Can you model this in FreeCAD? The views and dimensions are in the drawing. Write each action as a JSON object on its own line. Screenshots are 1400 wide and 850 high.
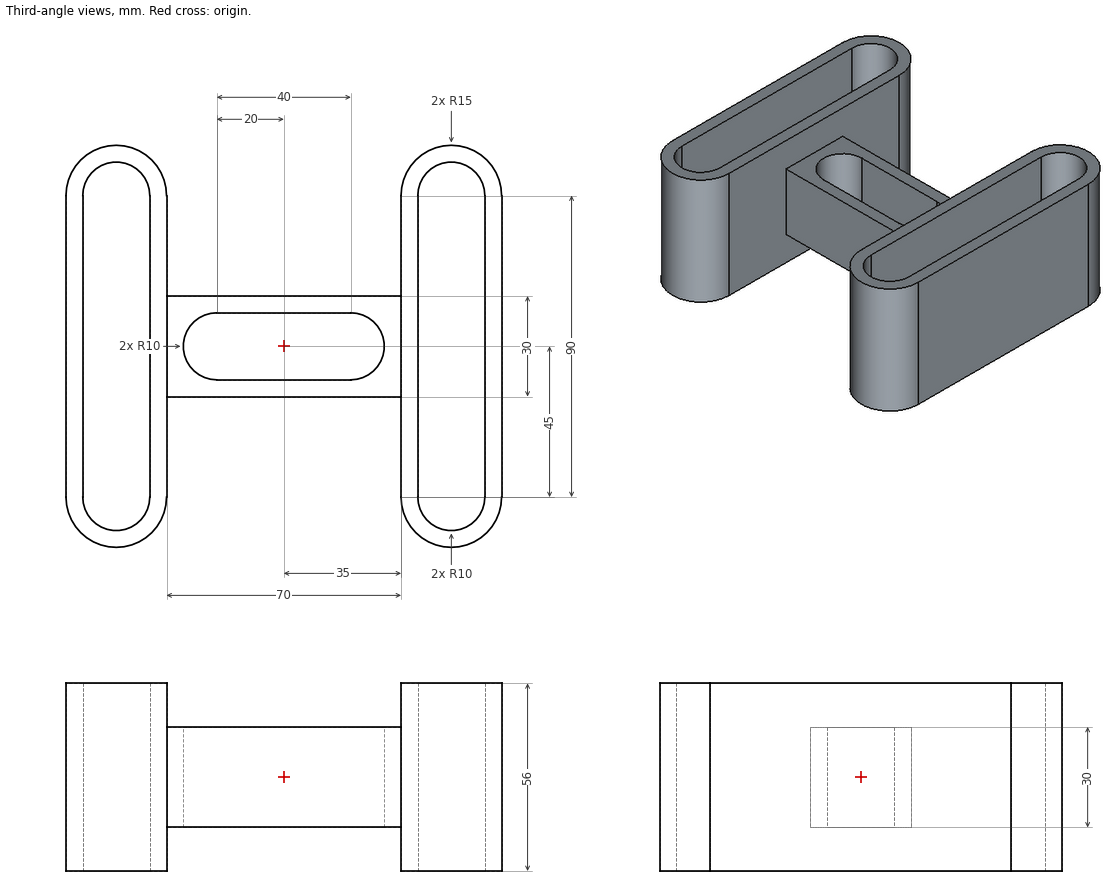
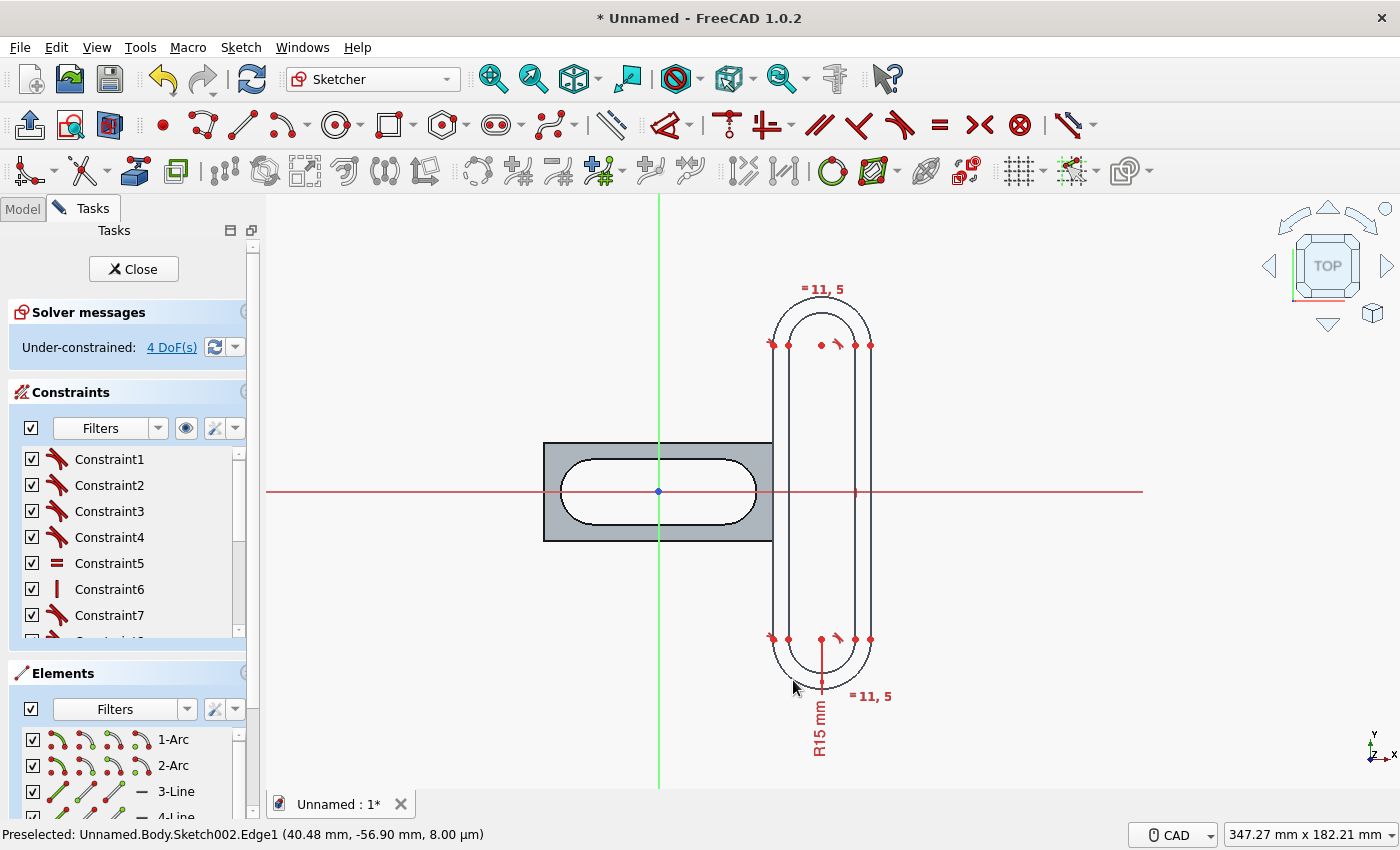
{"action": "left_click", "coordinate": [803, 667]}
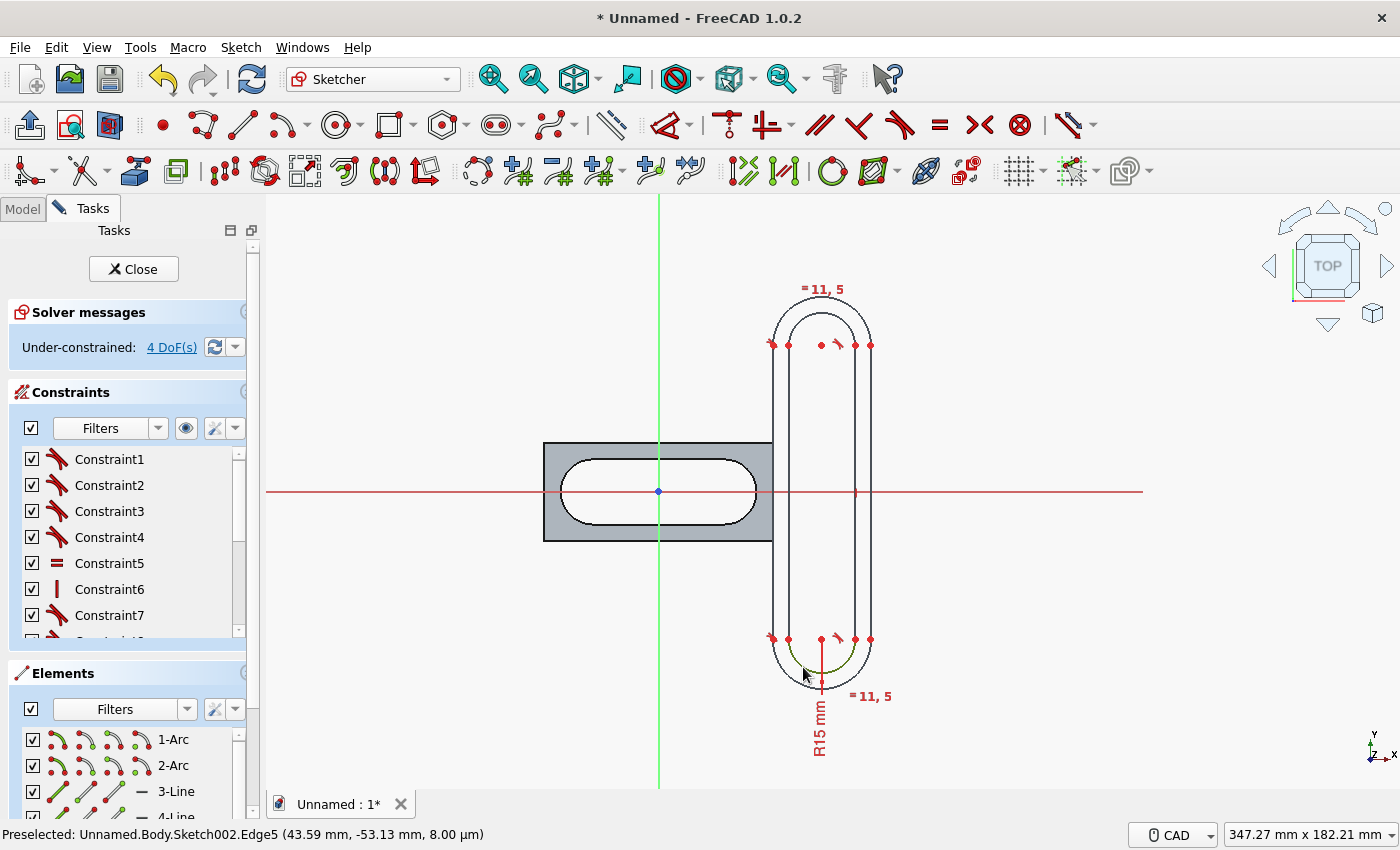
{"action": "key", "text": "k r"}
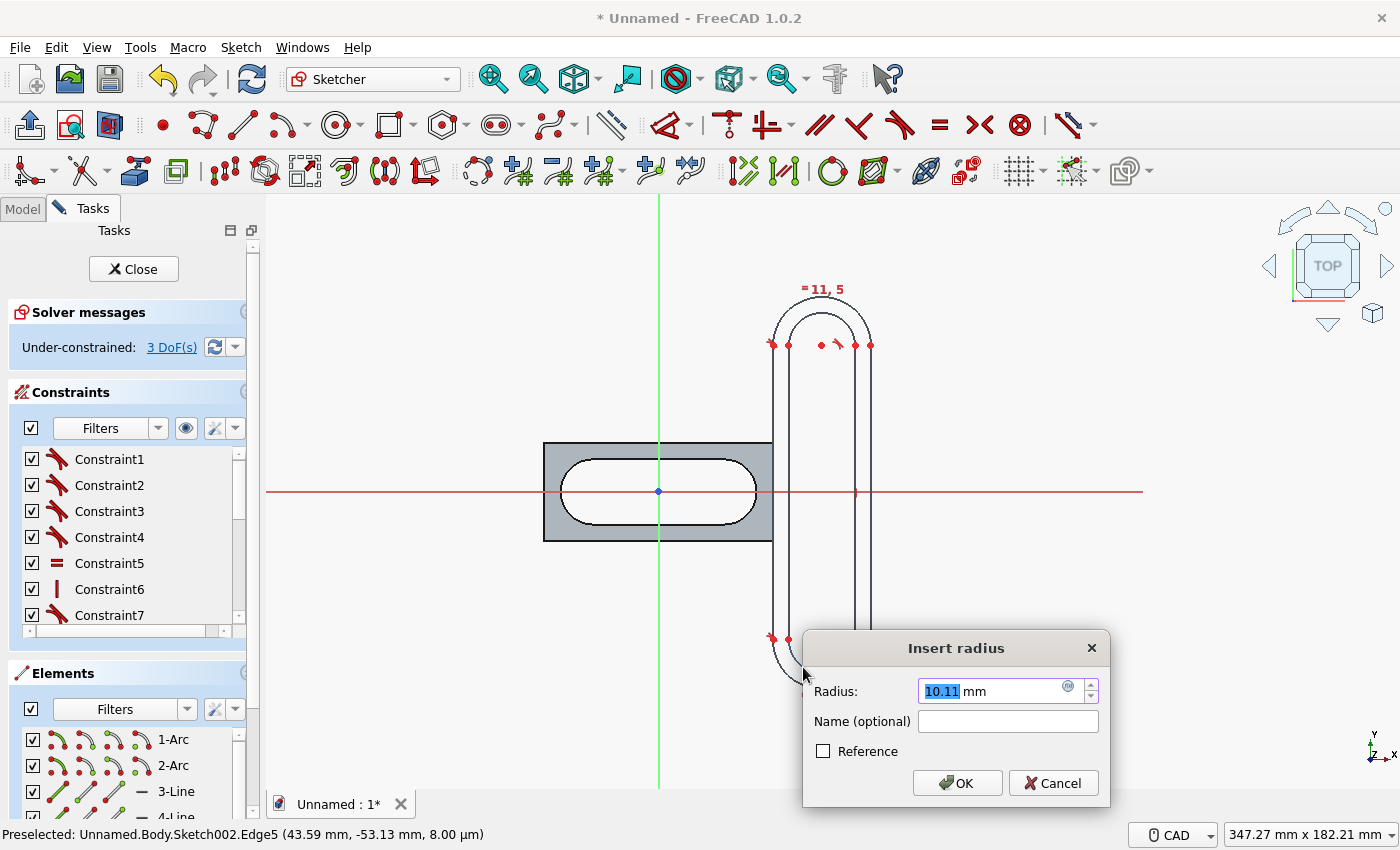
{"action": "type", "text": "10"}
{"action": "key", "text": "Return"}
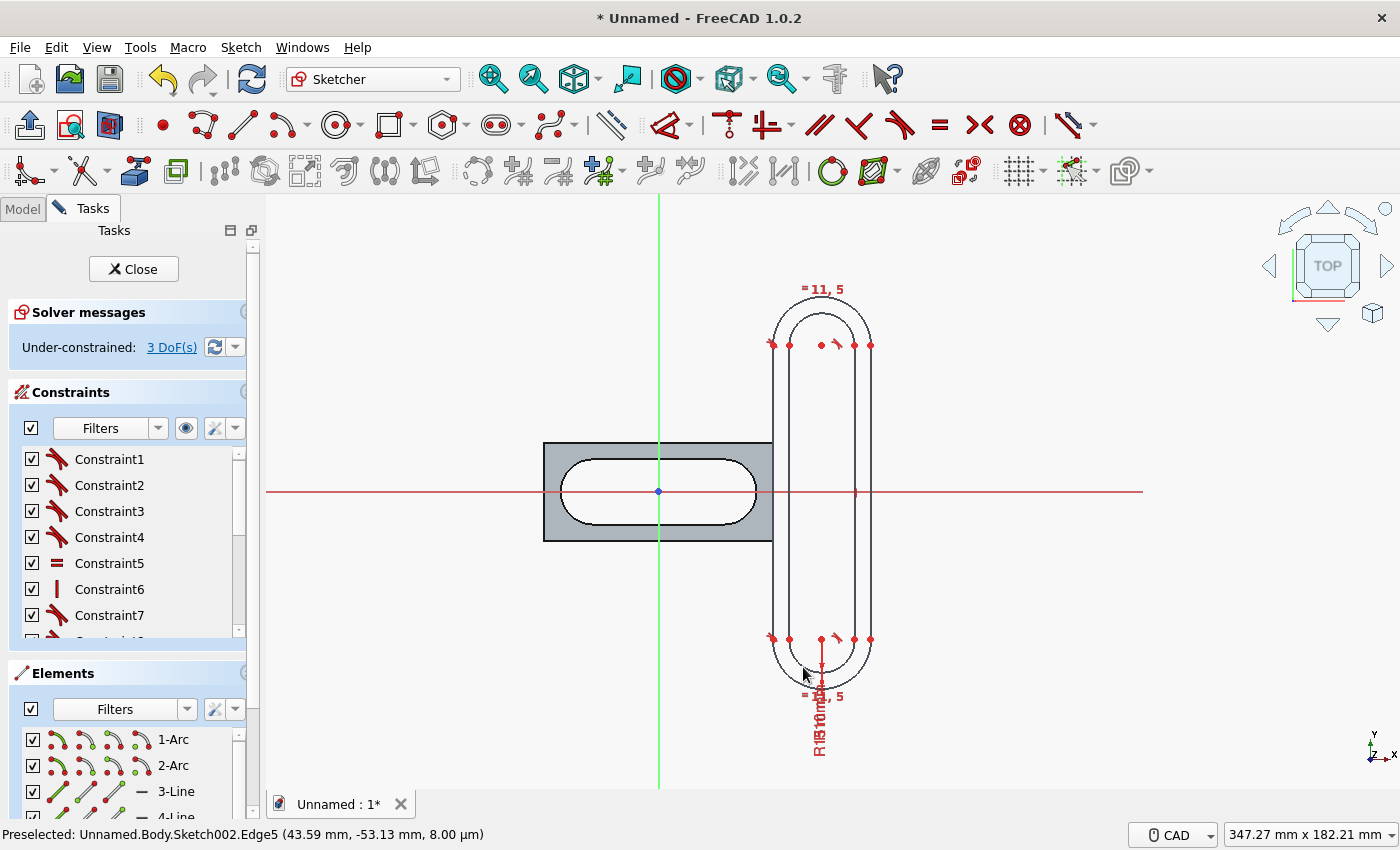
{"action": "left_click", "coordinate": [773, 552]}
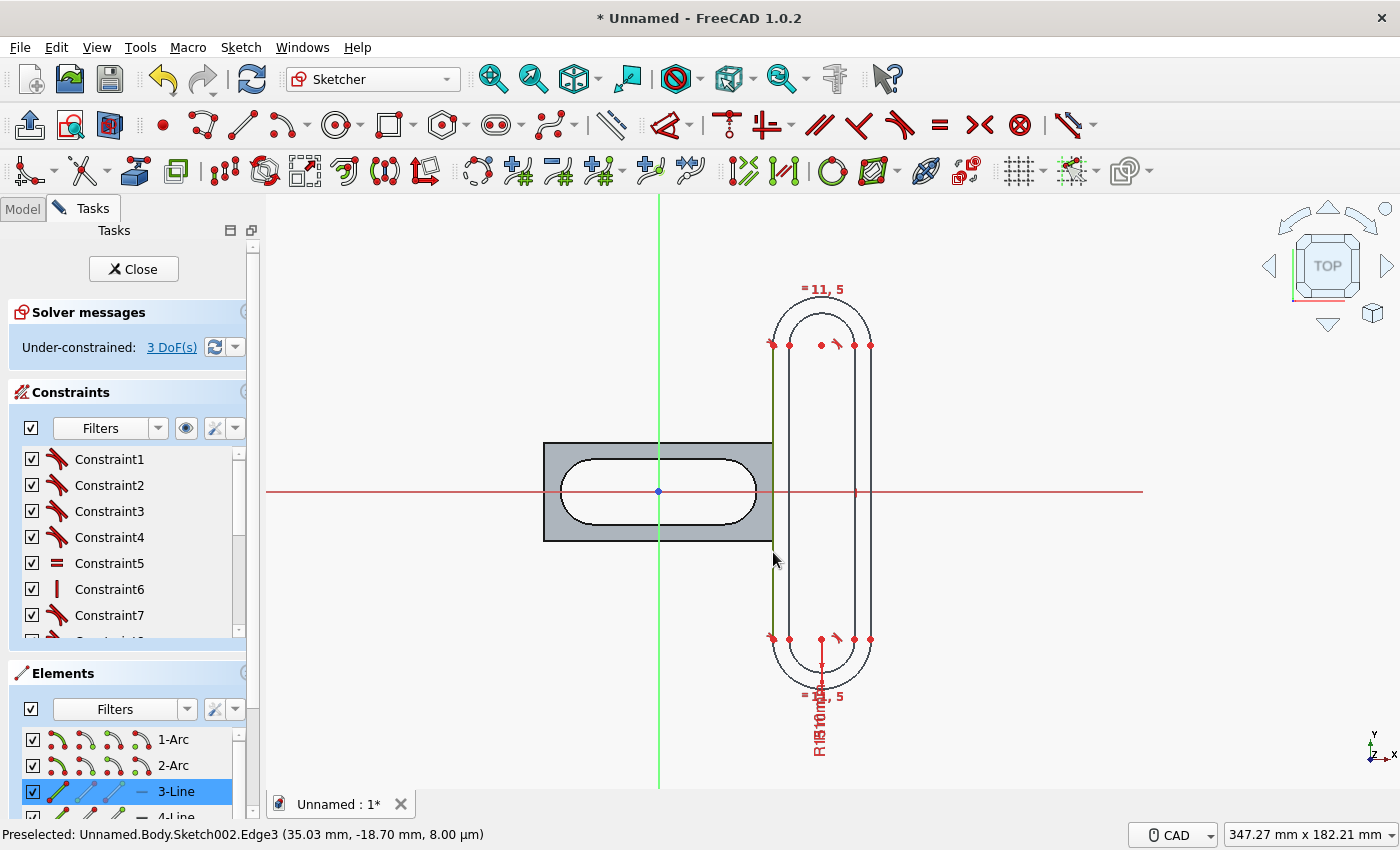
{"action": "key", "text": "i"}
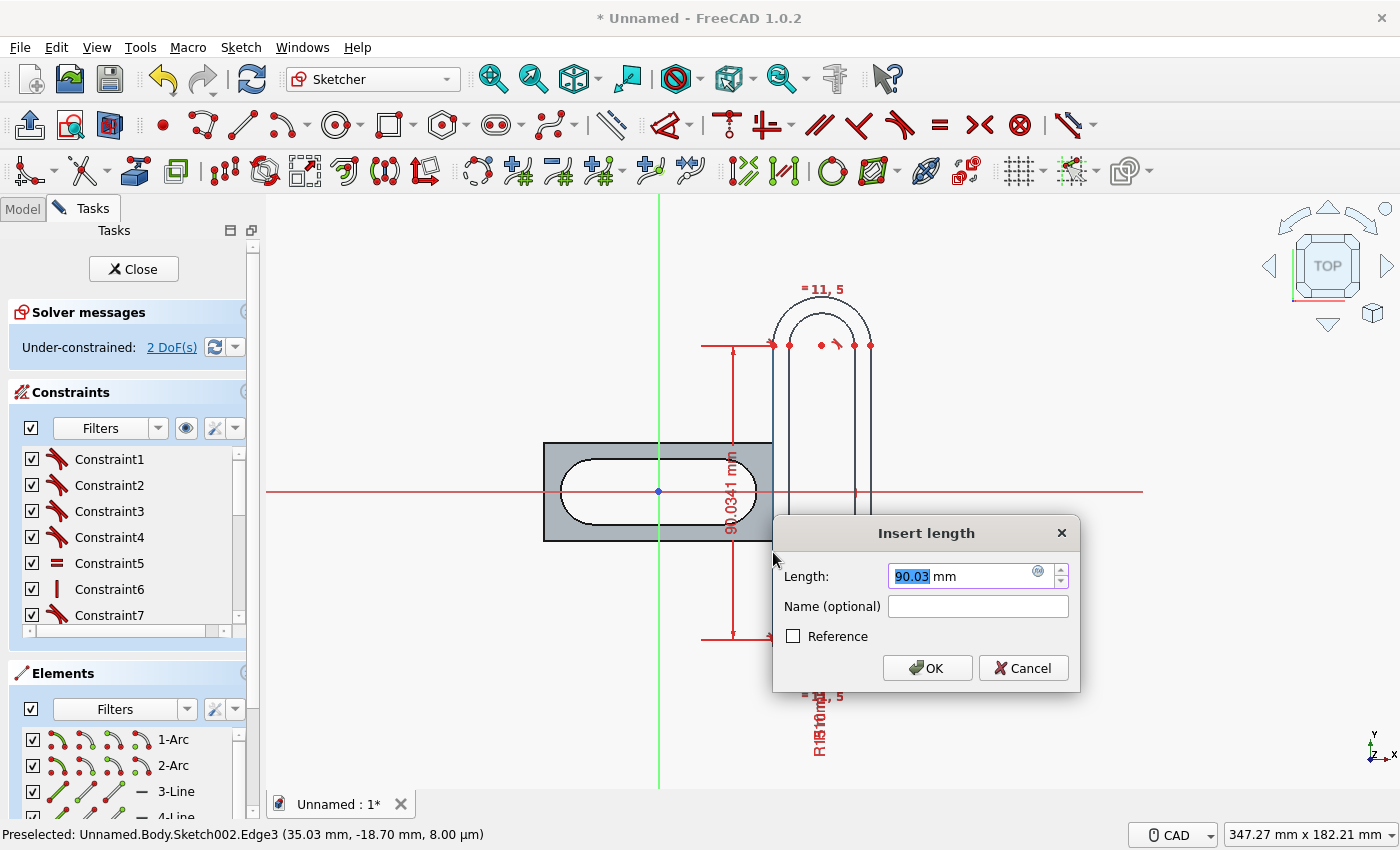
{"action": "type", "text": "90"}
{"action": "key", "text": "Return"}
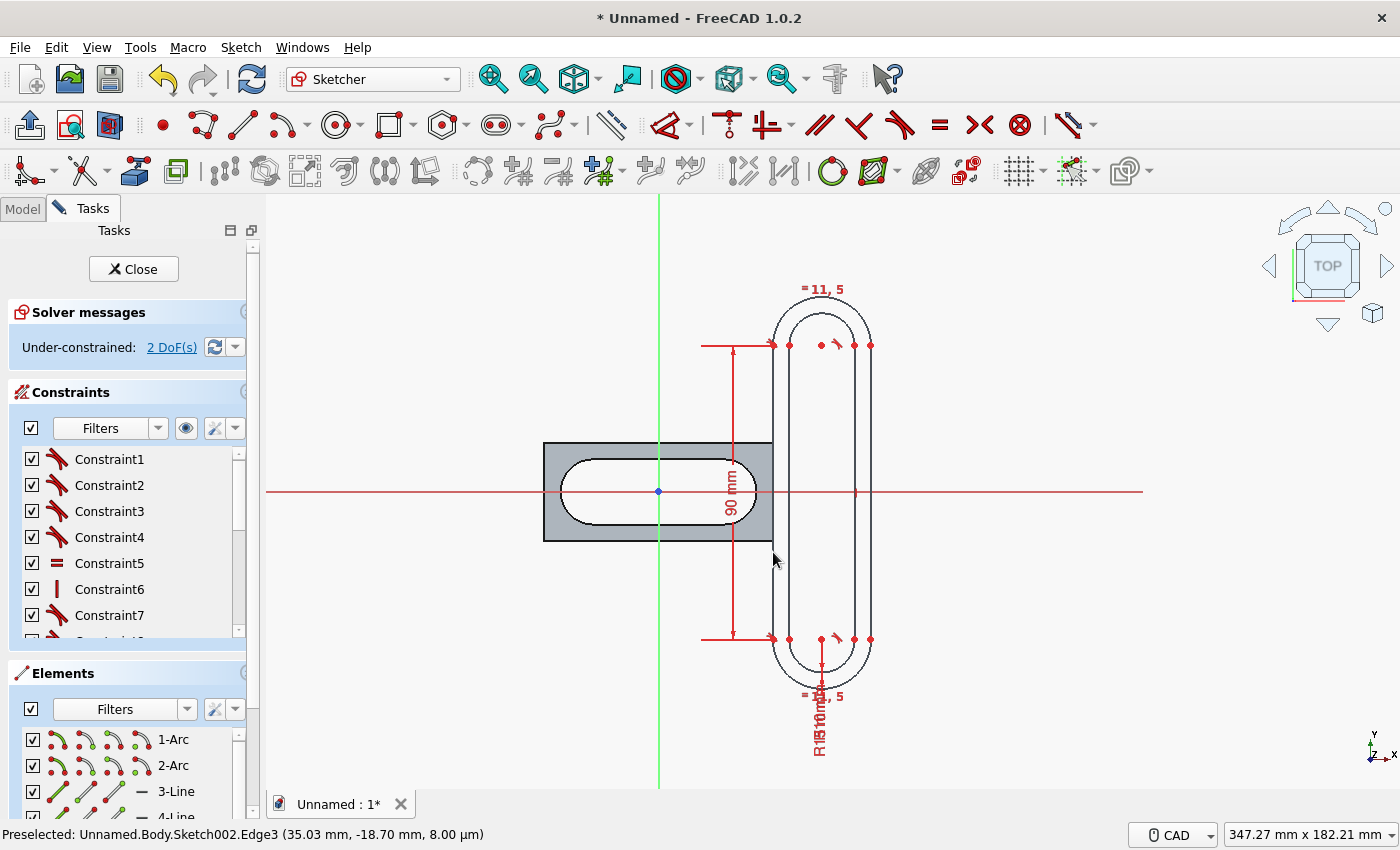
{"action": "left_click", "coordinate": [773, 640]}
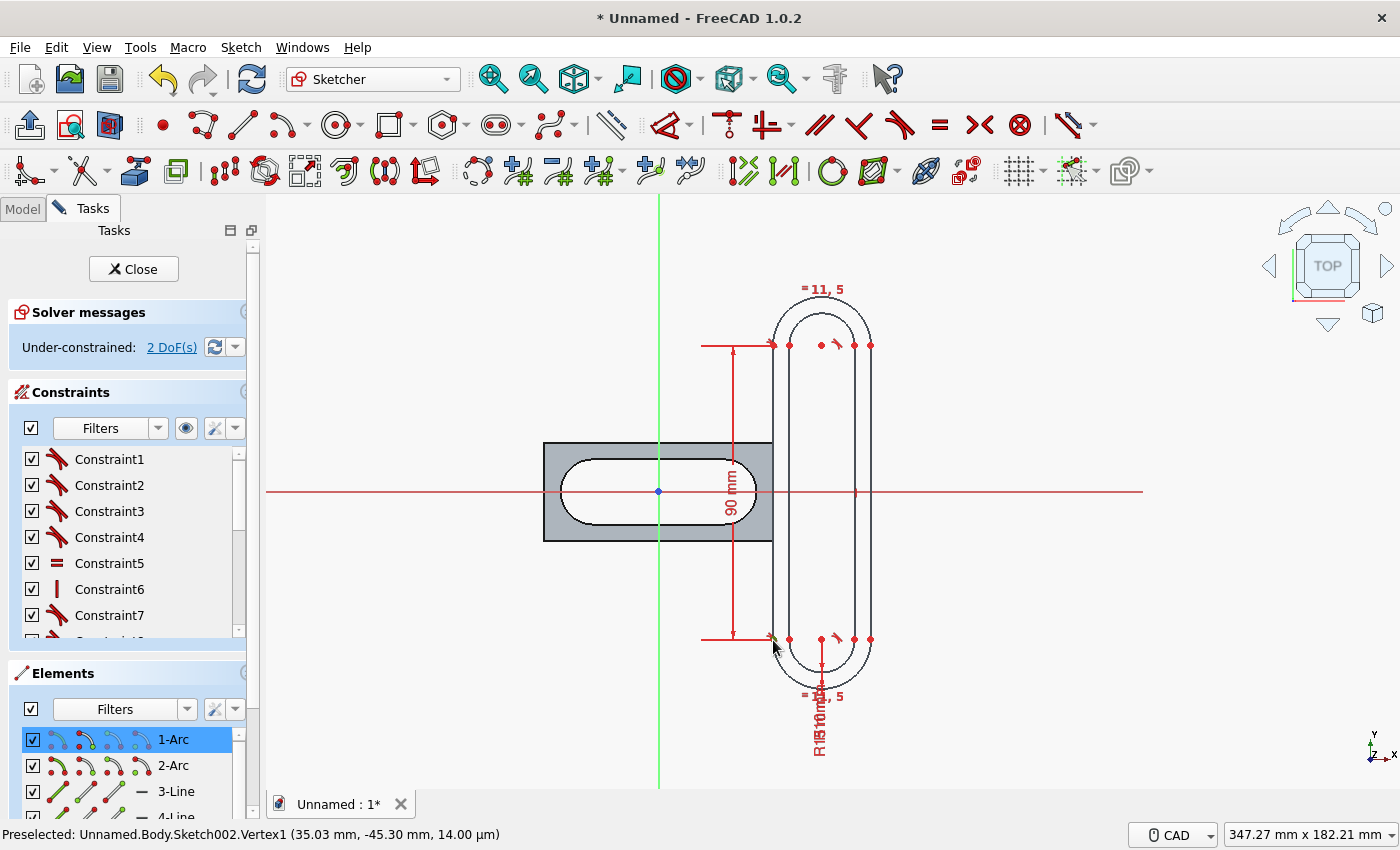
{"action": "key", "text": "l"}